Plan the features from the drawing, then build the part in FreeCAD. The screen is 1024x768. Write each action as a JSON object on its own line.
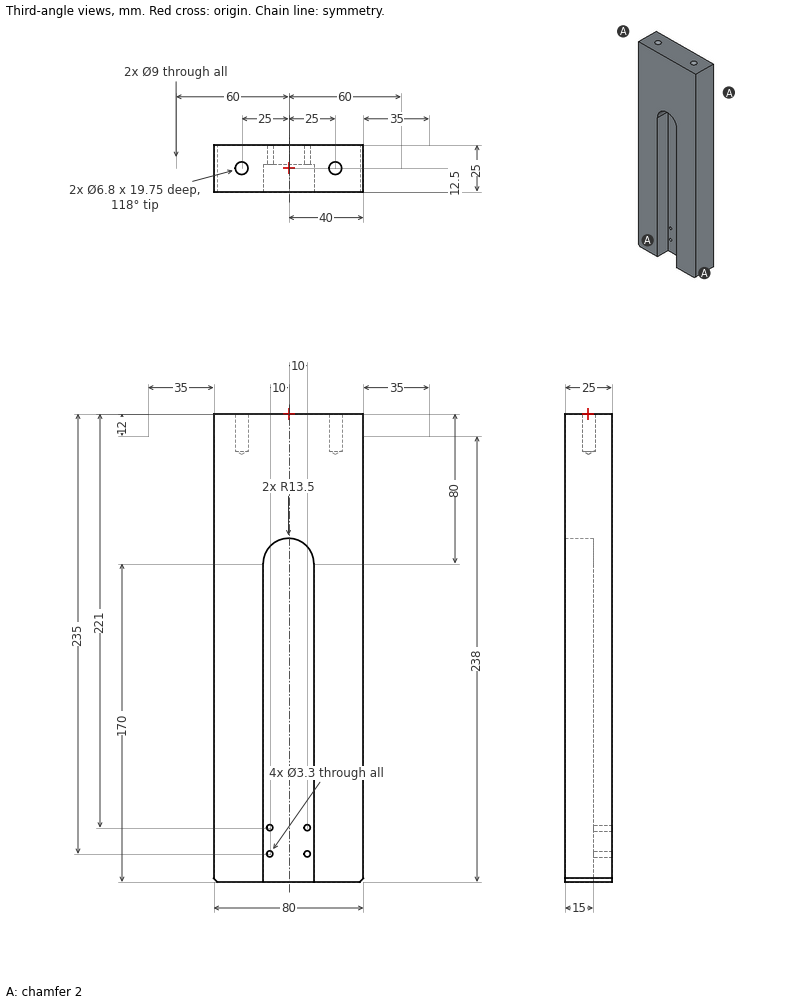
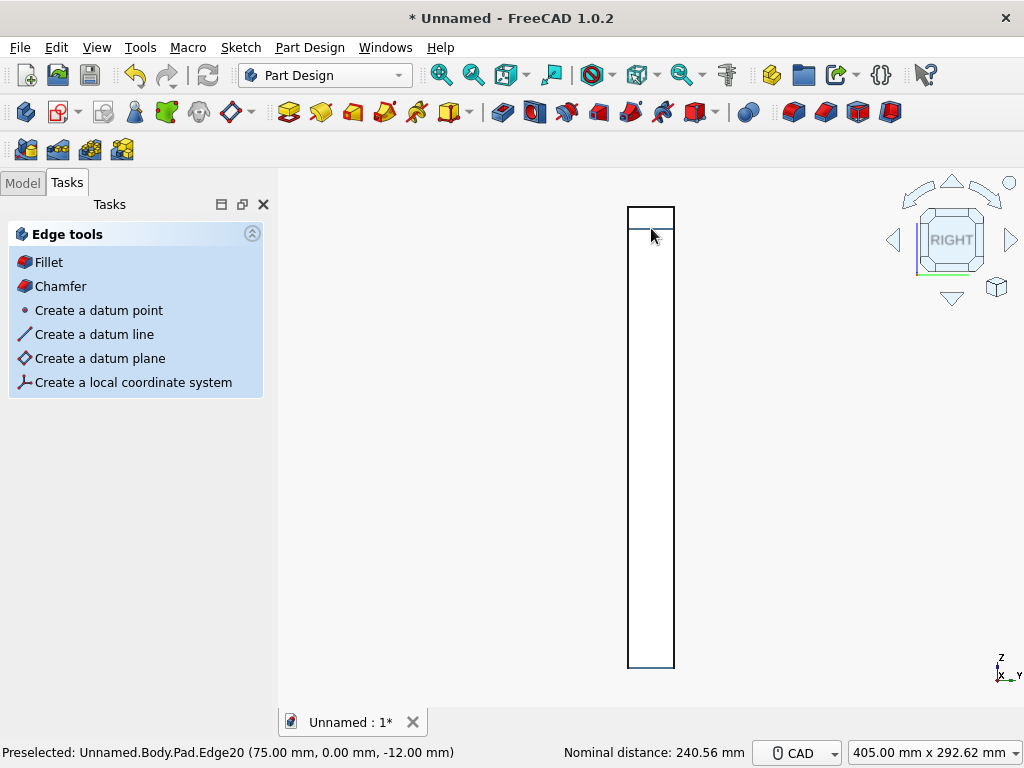
{"action": "key", "text": "5"}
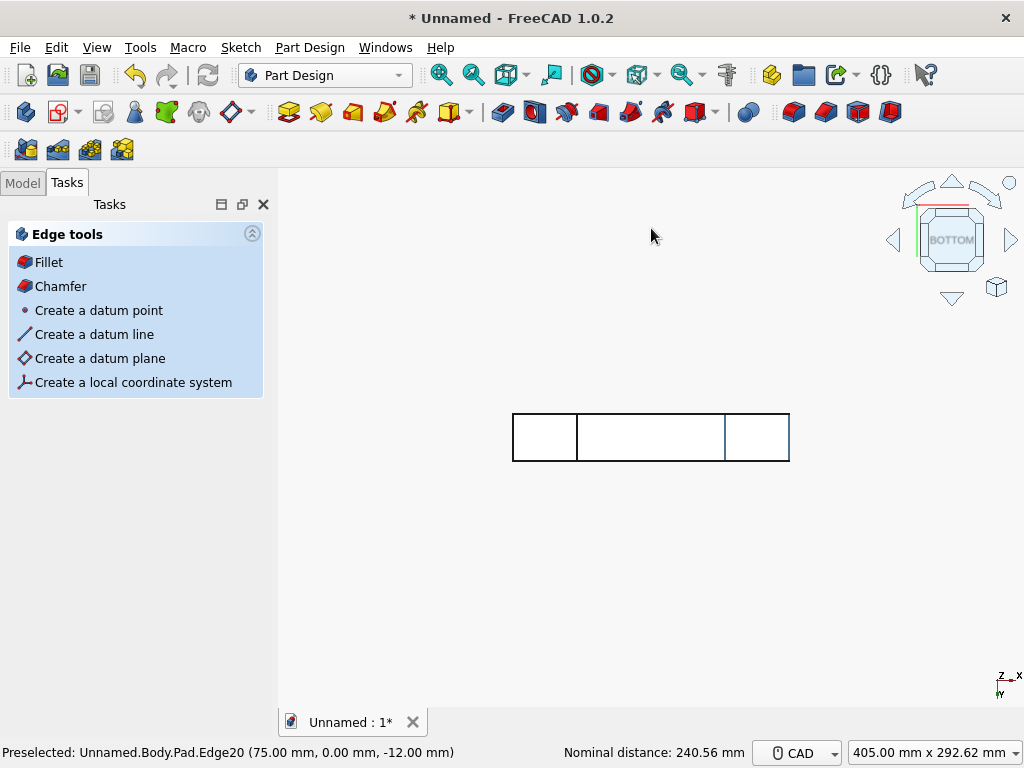
{"action": "left_click", "coordinate": [442, 76]}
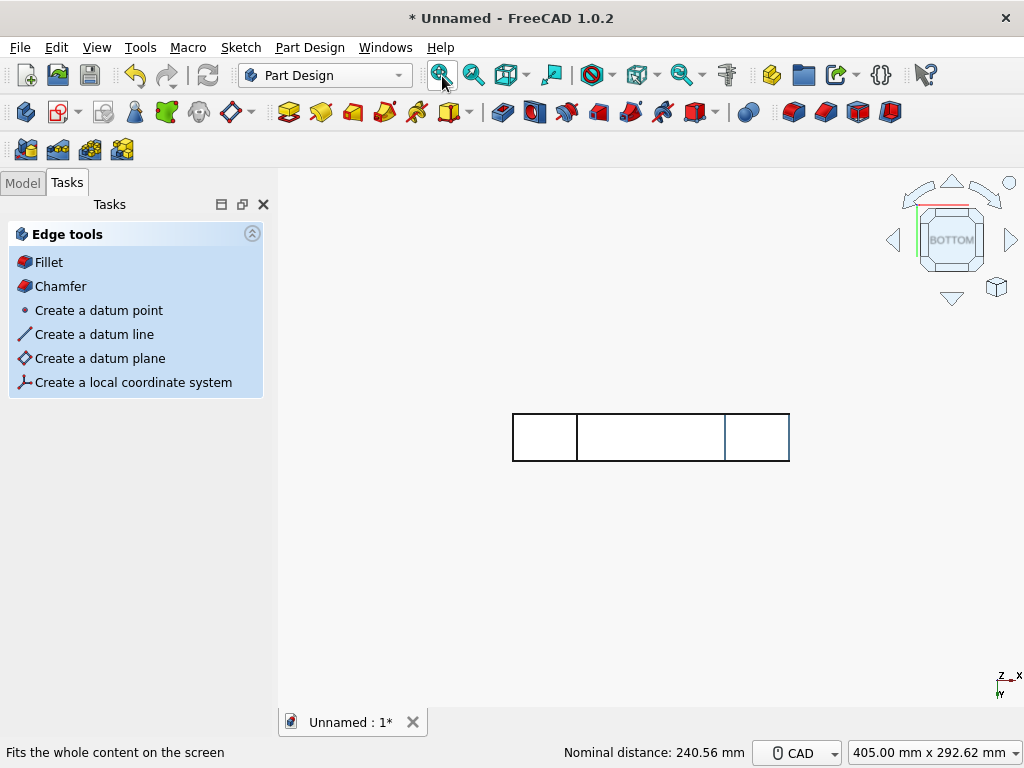
{"action": "left_click", "coordinate": [513, 436], "text": "ctrl"}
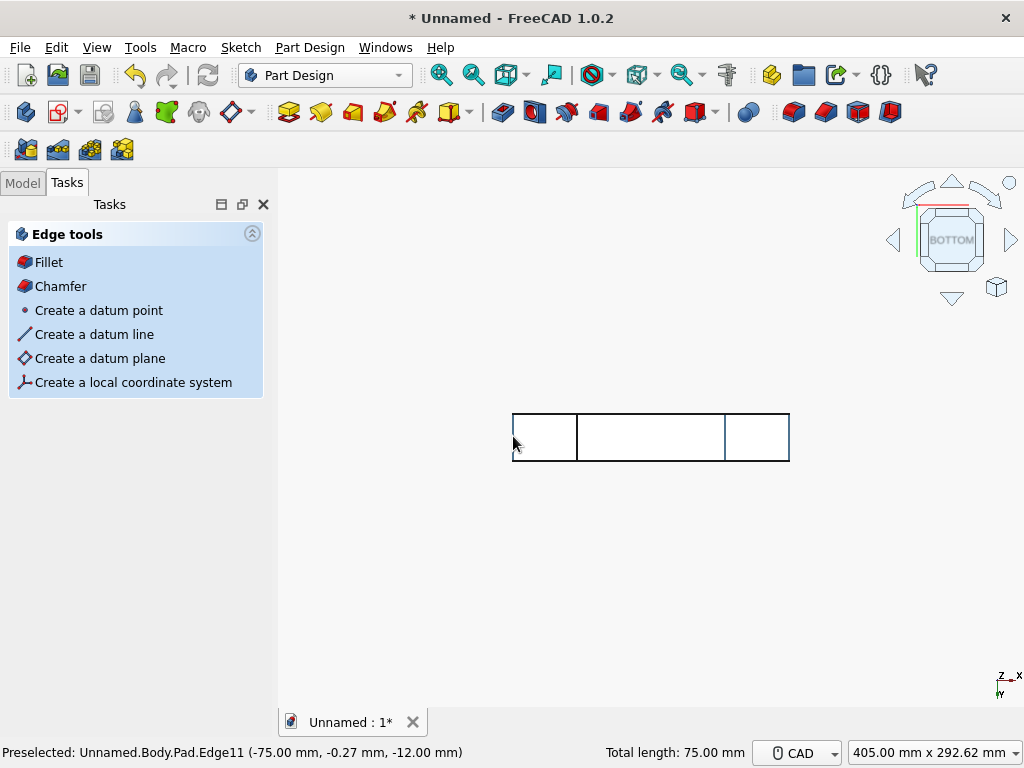
{"action": "left_click", "coordinate": [577, 436], "text": "ctrl"}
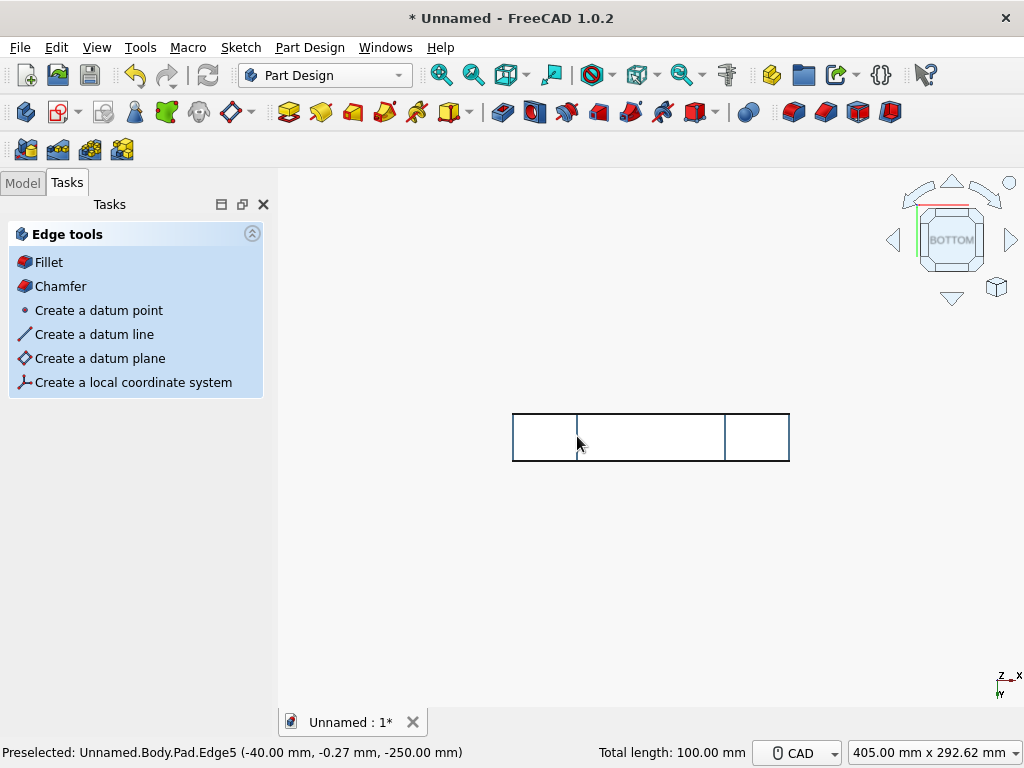
{"action": "left_click", "coordinate": [826, 112]}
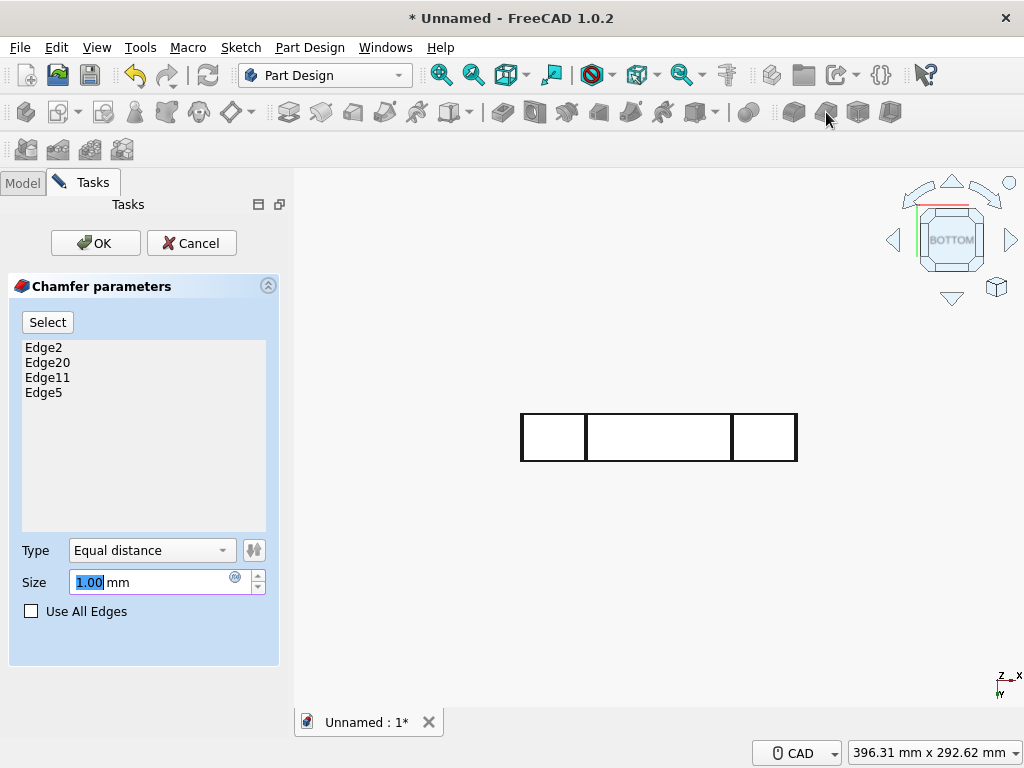
{"action": "type", "text": "2"}
{"action": "key", "text": "Tab"}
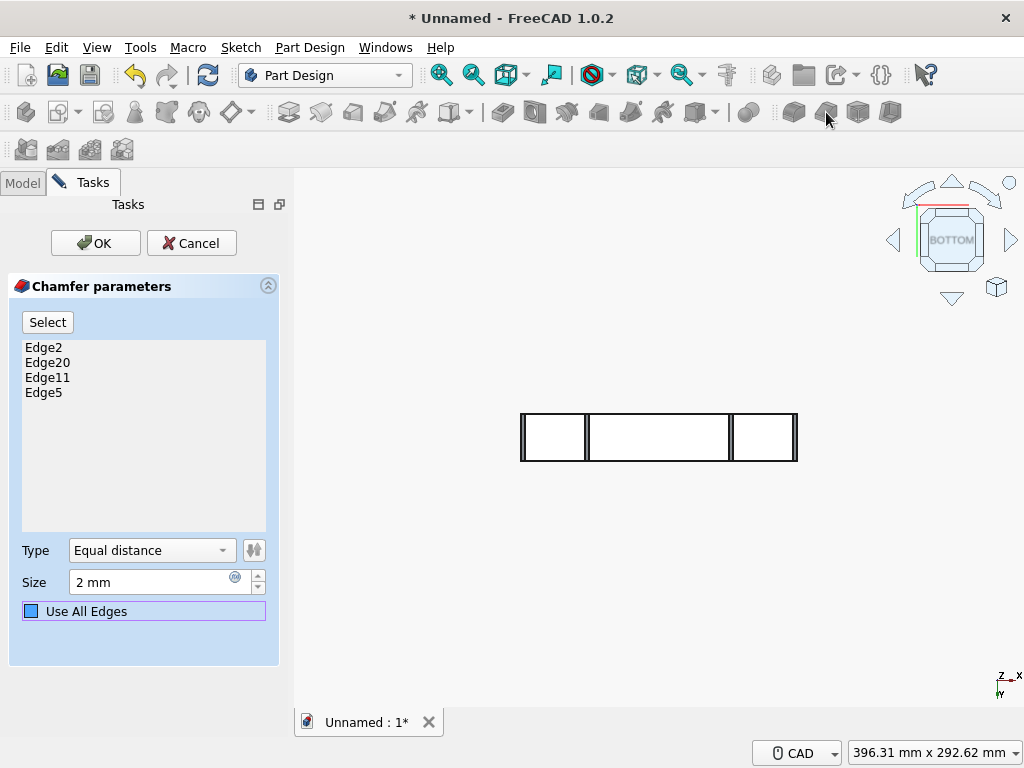
{"action": "left_click", "coordinate": [96, 243]}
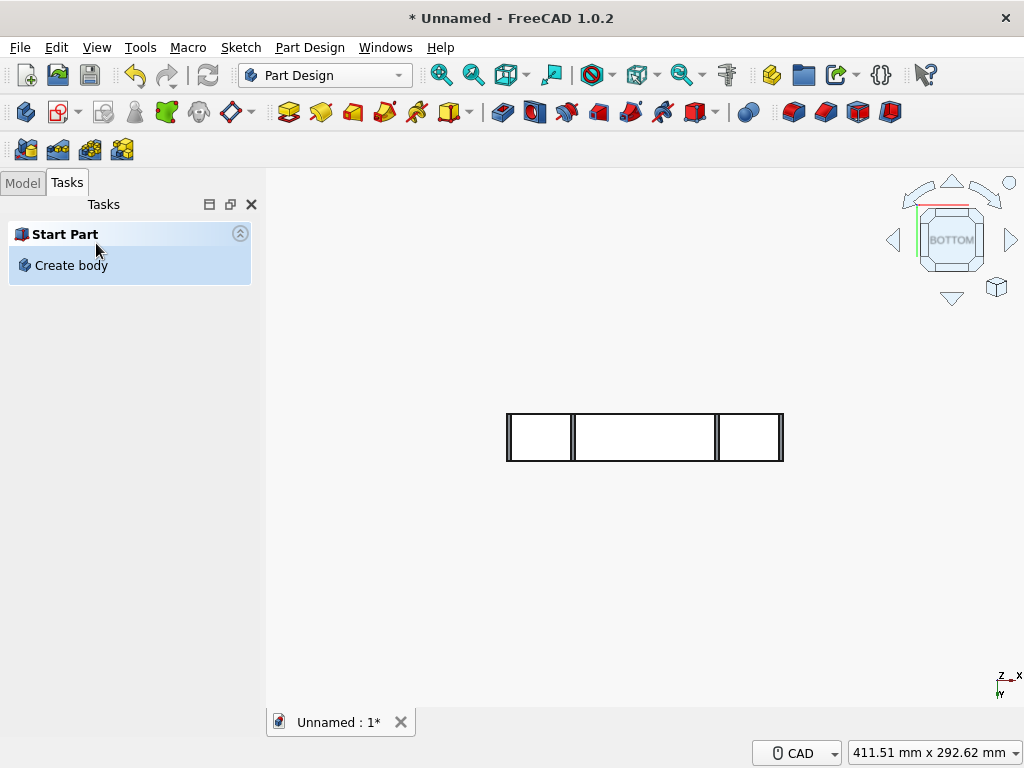
{"action": "left_click", "coordinate": [442, 76]}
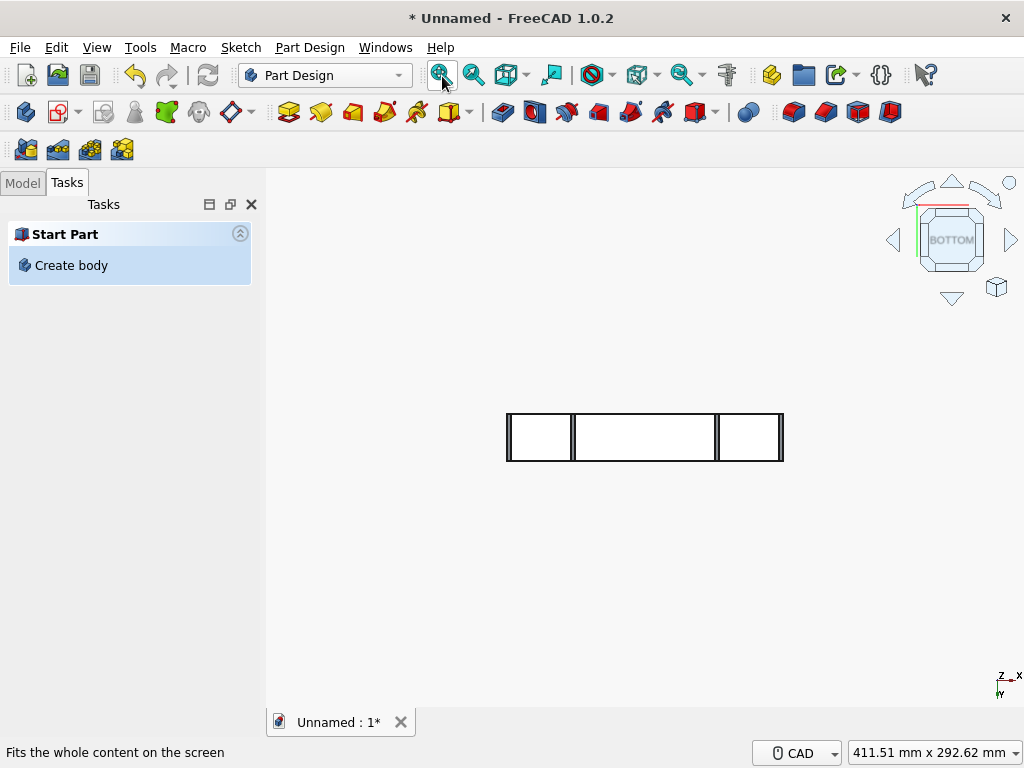
{"action": "left_click", "coordinate": [58, 112]}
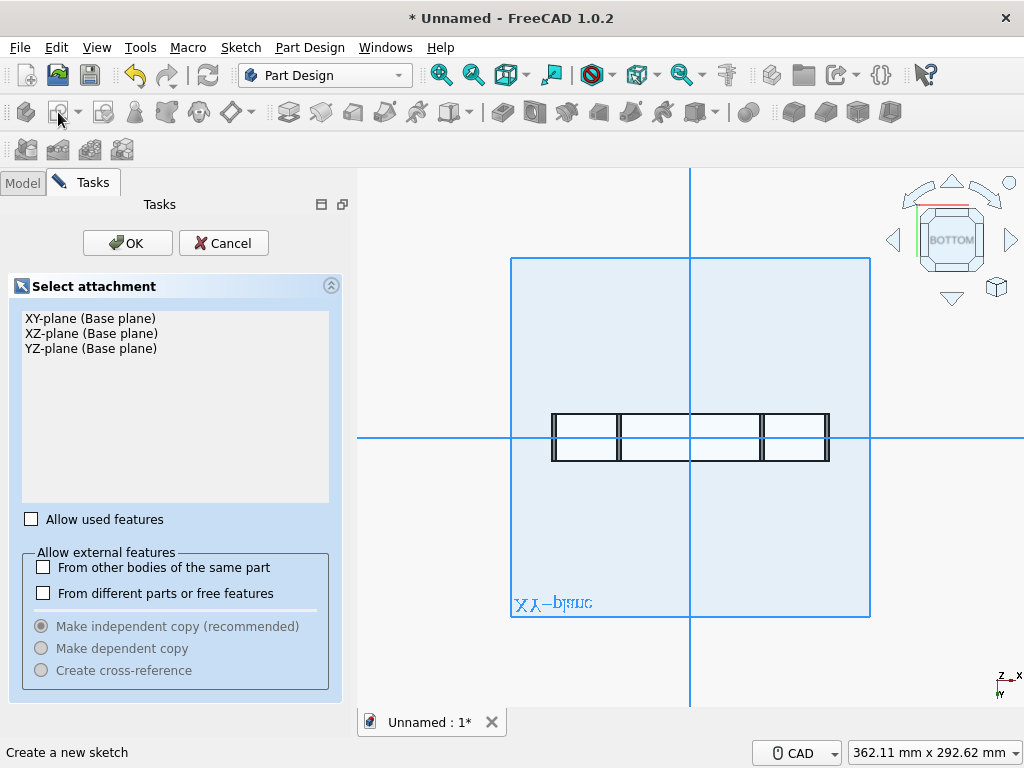
{"action": "left_click", "coordinate": [82, 318]}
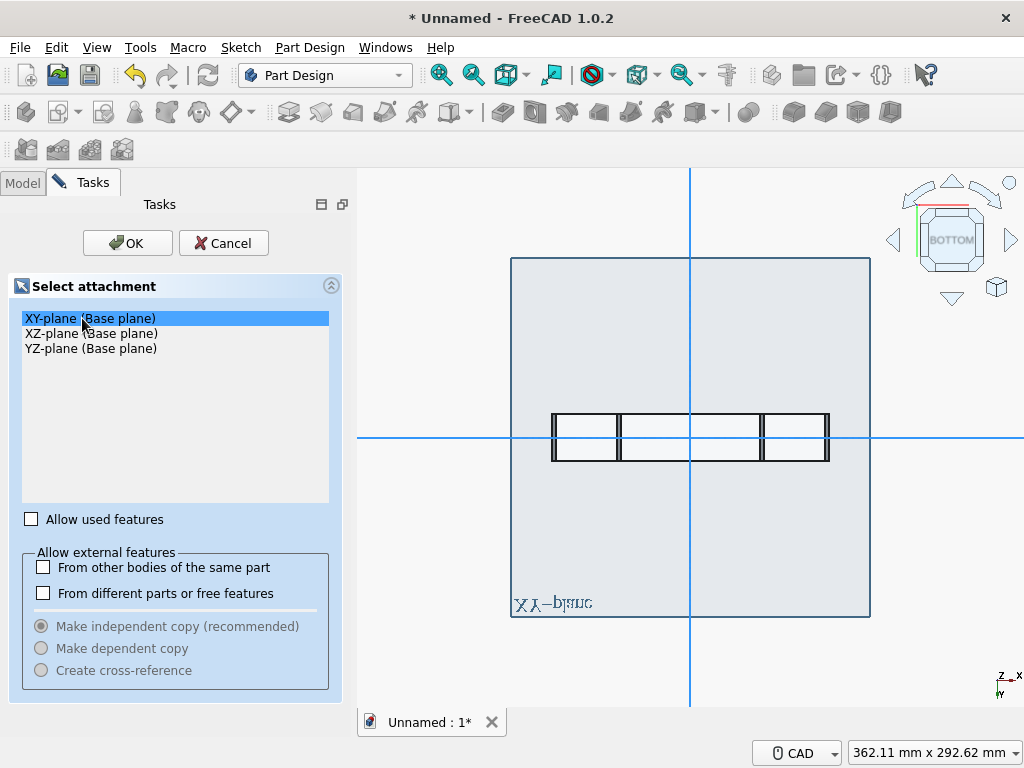
{"action": "left_click", "coordinate": [128, 243]}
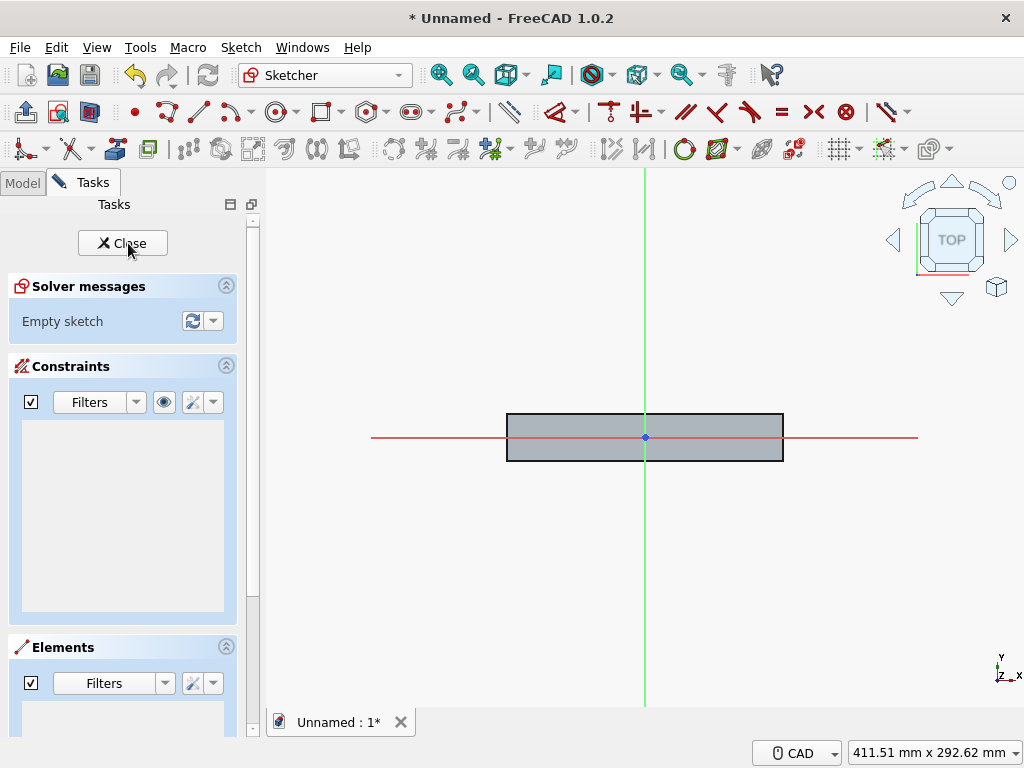
{"action": "scroll", "coordinate": [728, 438], "scroll_direction": "up", "scroll_amount": 3}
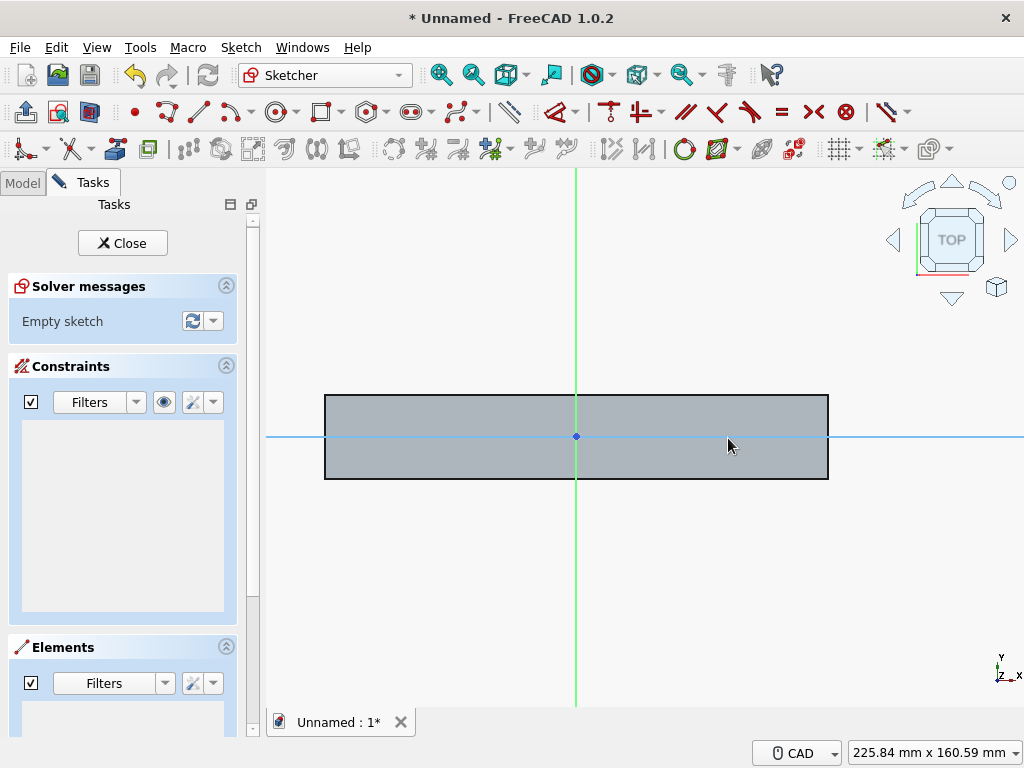
{"action": "left_click", "coordinate": [276, 112]}